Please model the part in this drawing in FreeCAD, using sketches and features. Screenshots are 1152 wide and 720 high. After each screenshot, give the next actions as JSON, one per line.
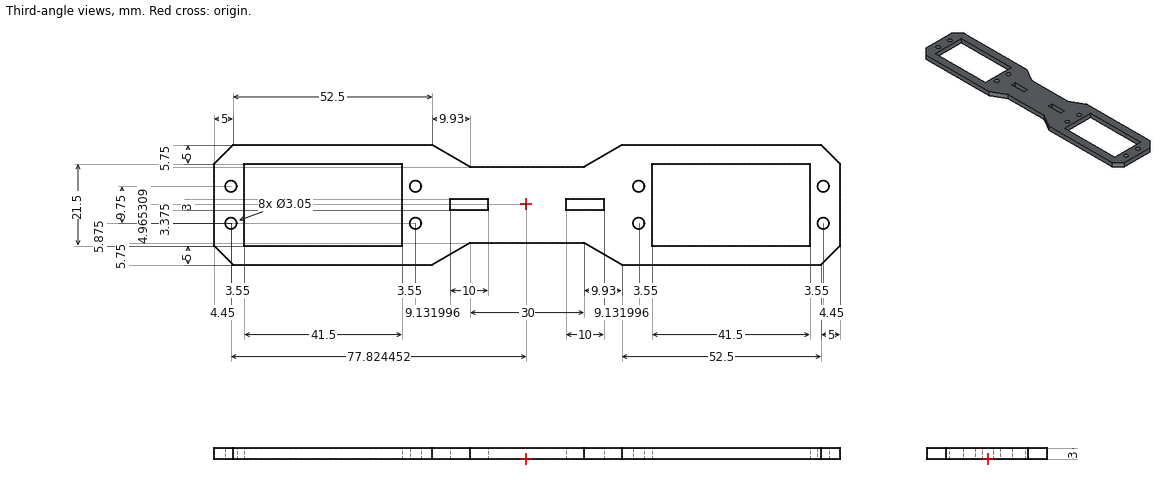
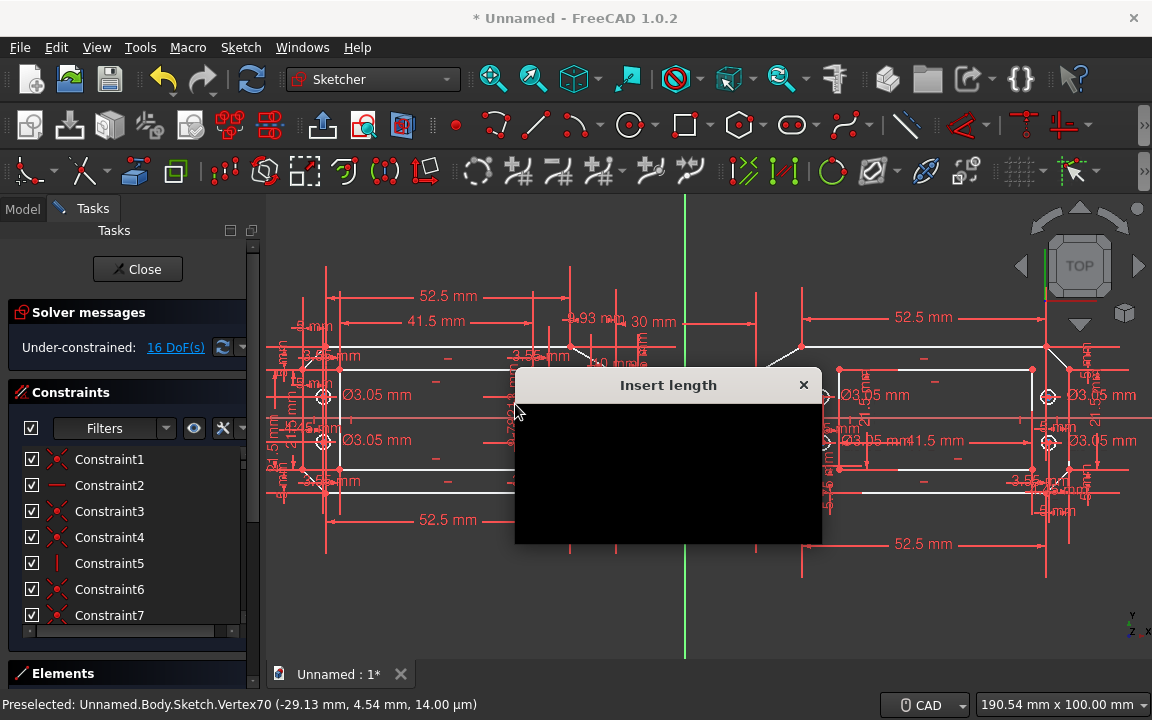
{"action": "type", "text": "9.75"}
{"action": "key", "text": "Return"}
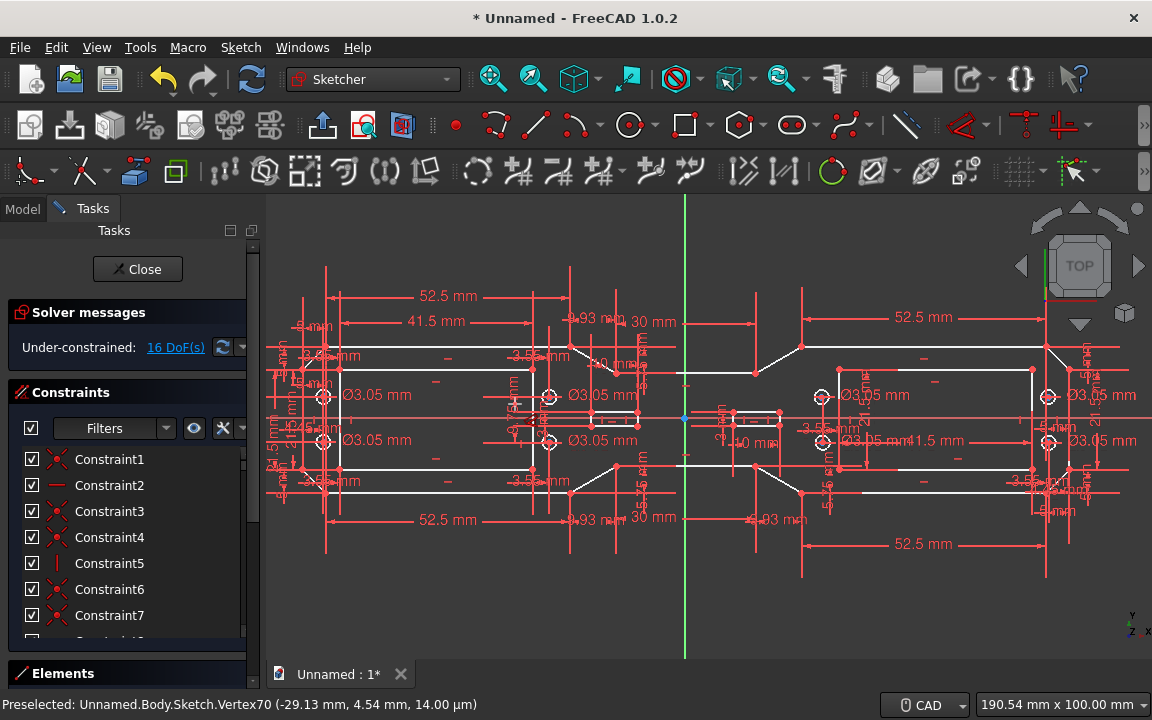
{"action": "scroll", "coordinate": [839, 370], "scroll_direction": "up", "scroll_amount": 5}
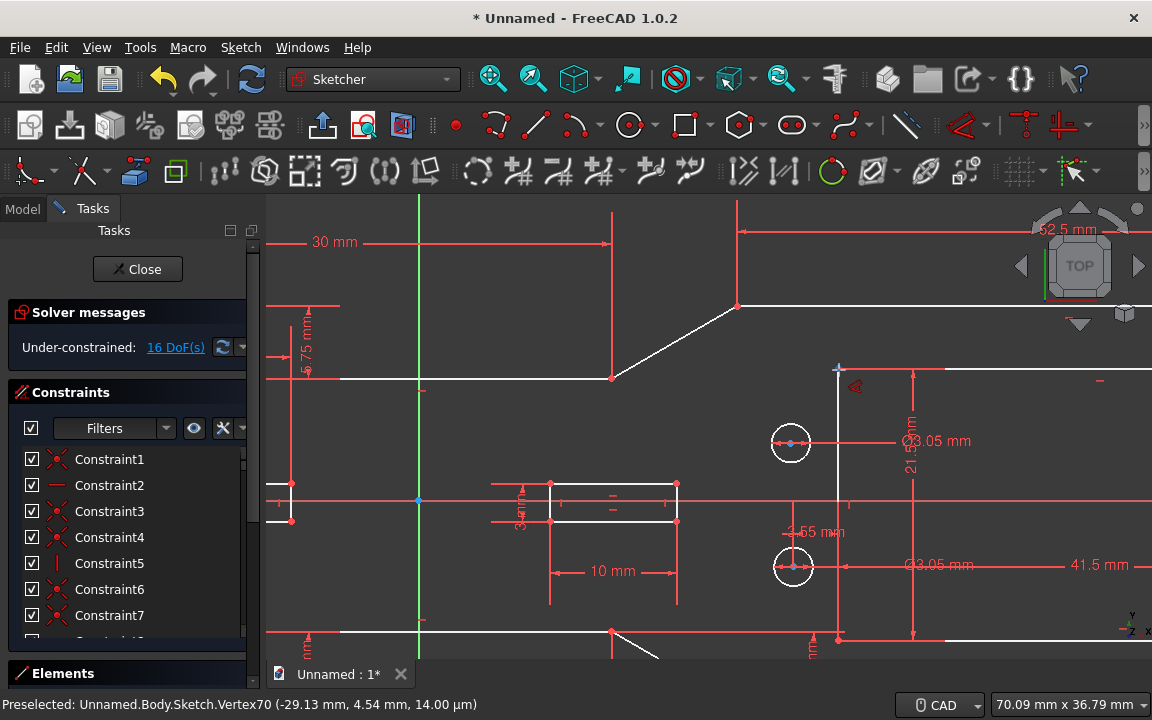
{"action": "left_click", "coordinate": [838, 369]}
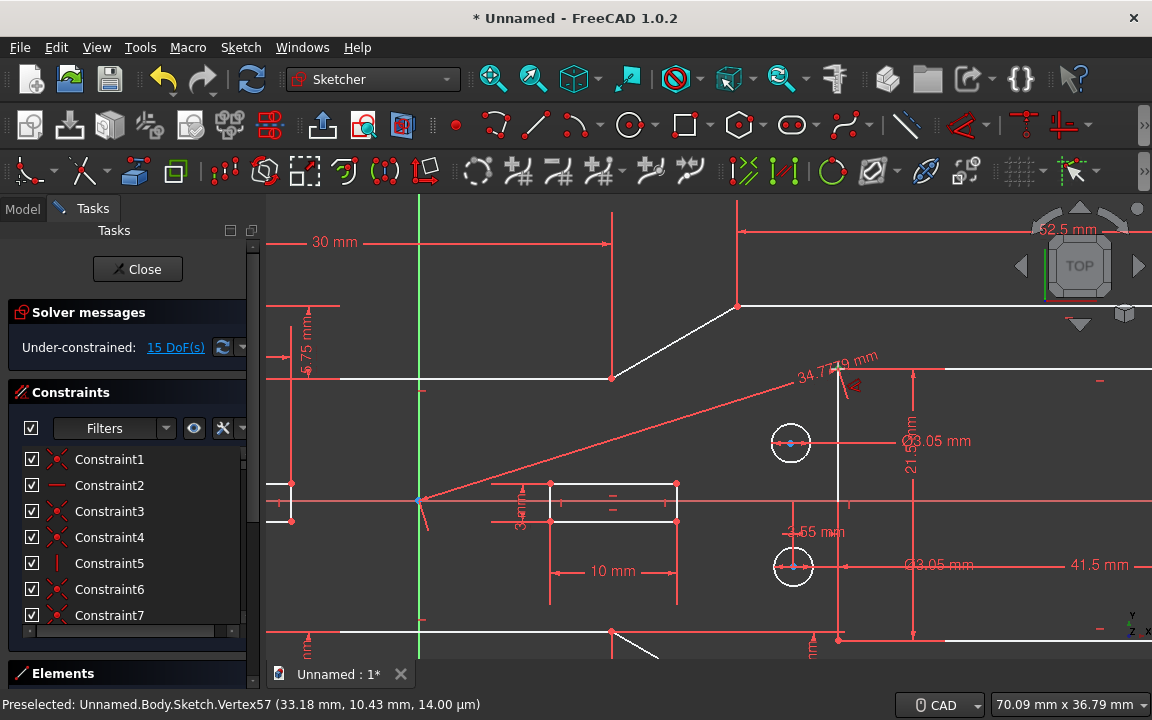
{"action": "left_click", "coordinate": [791, 443]}
{"action": "left_click", "coordinate": [815, 335]}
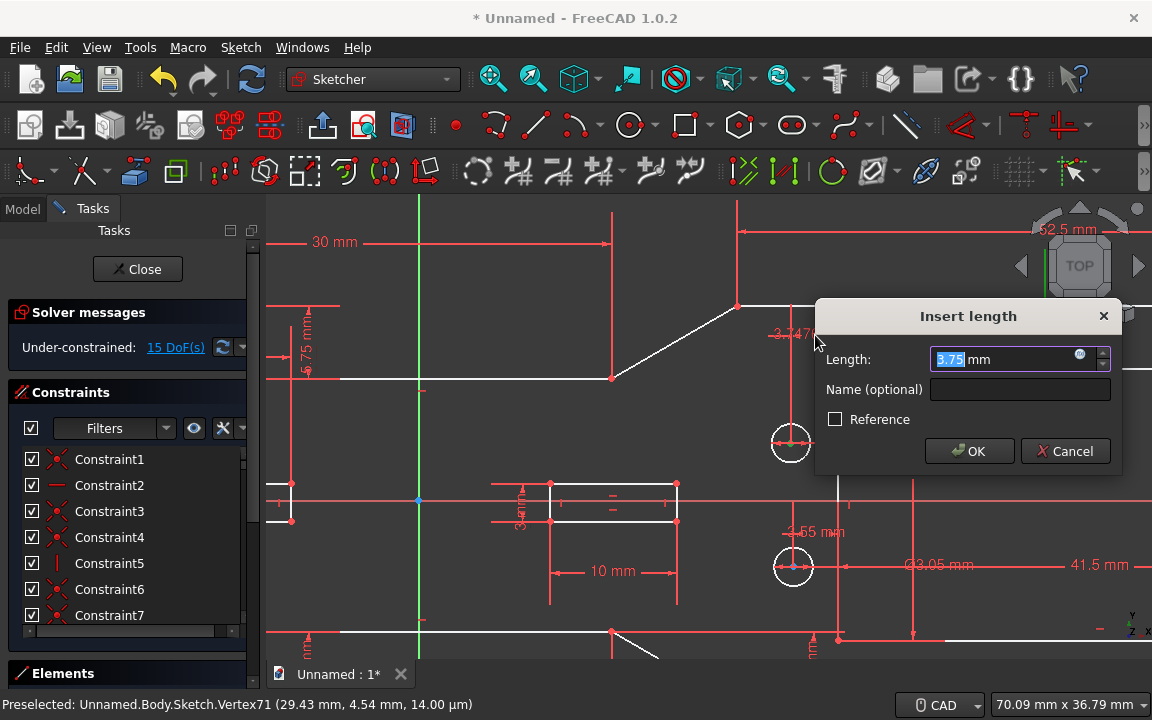
{"action": "type", "text": "3.55"}
{"action": "key", "text": "Return"}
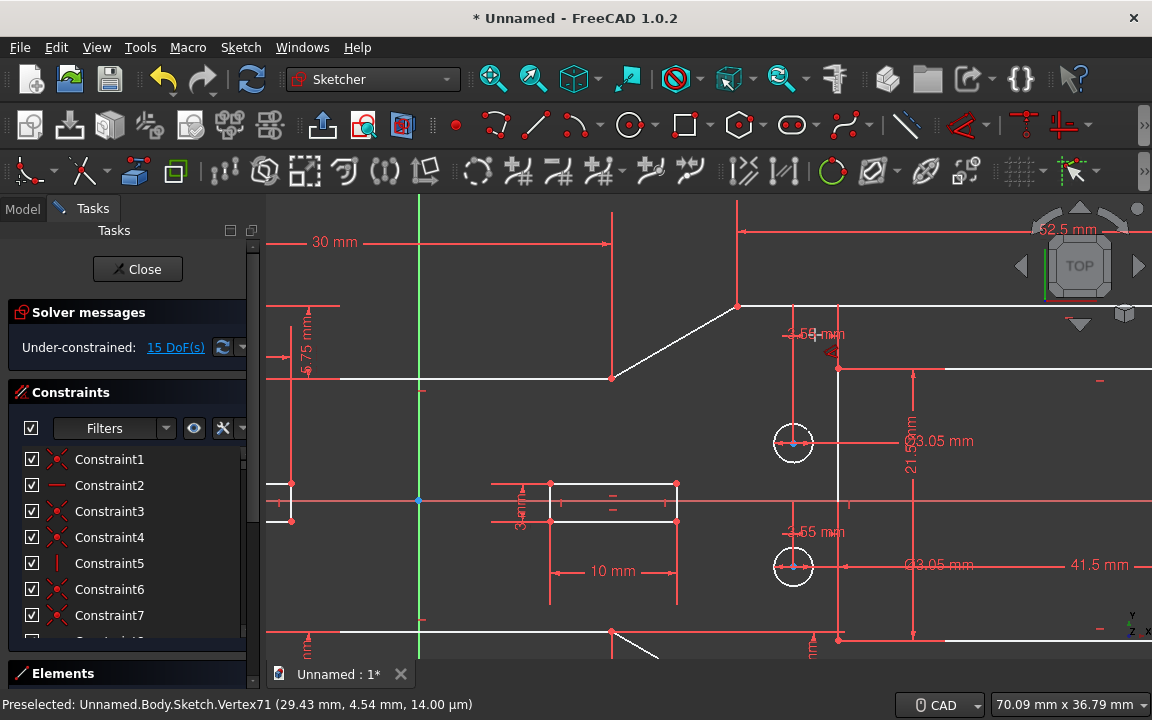
{"action": "scroll", "coordinate": [712, 402], "scroll_direction": "down", "scroll_amount": 7}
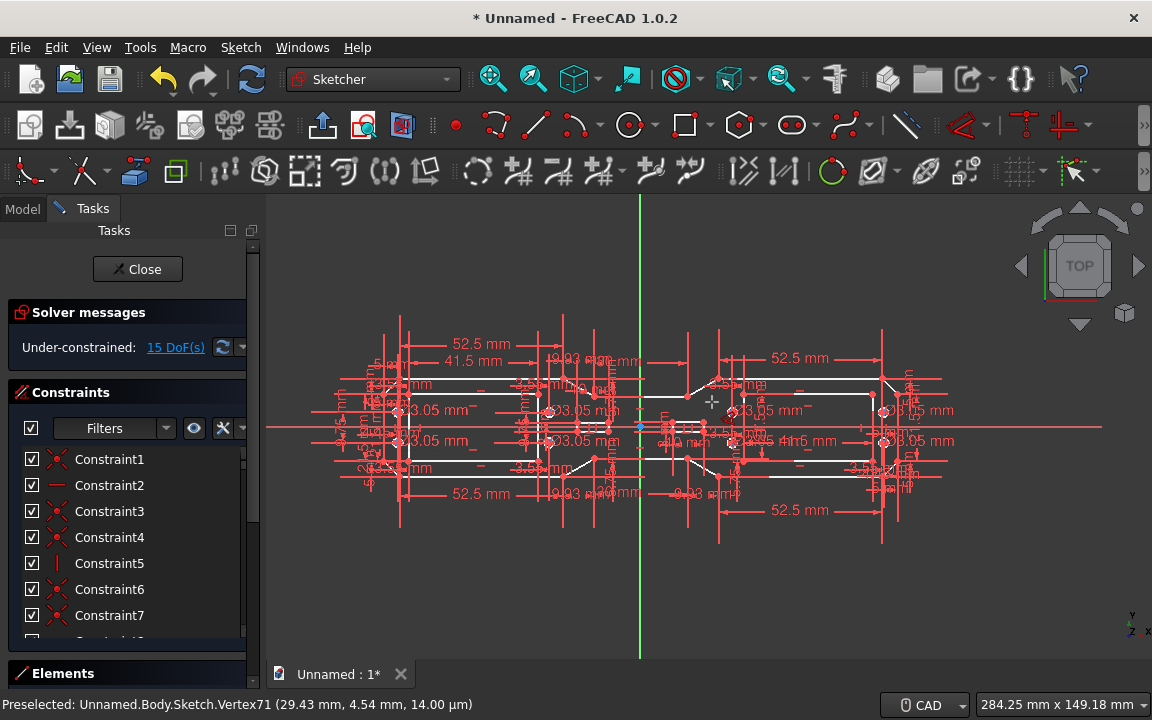
{"action": "scroll", "coordinate": [732, 443], "scroll_direction": "up", "scroll_amount": 2}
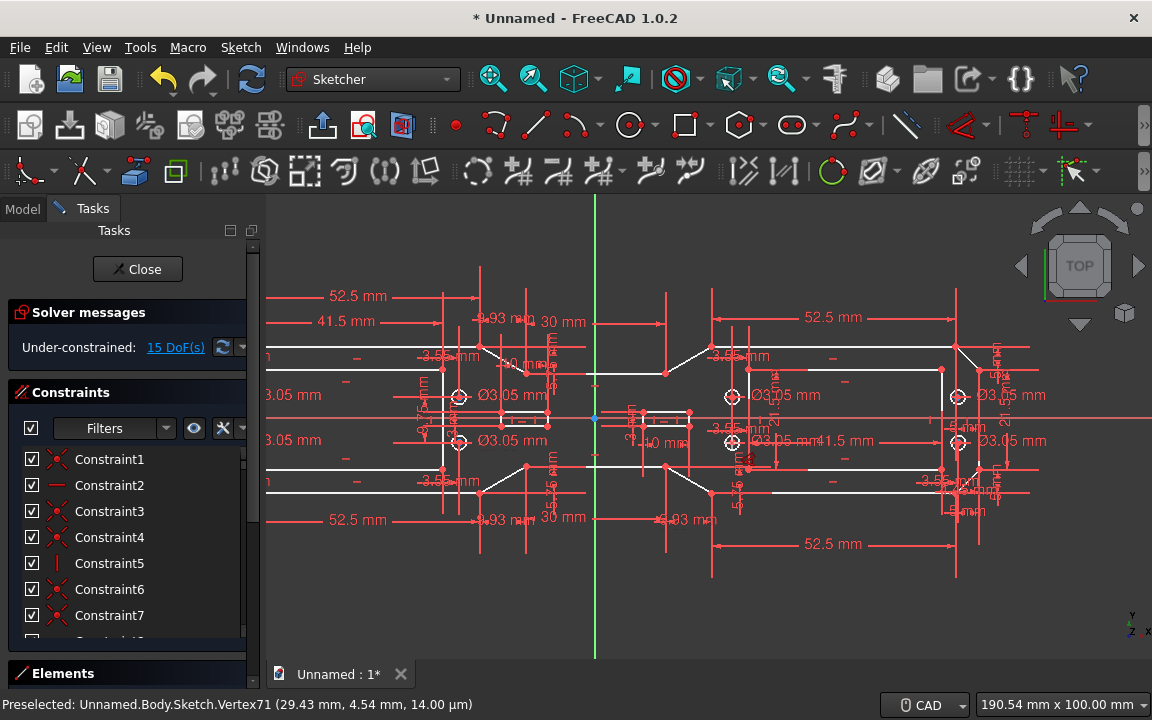
{"action": "left_click", "coordinate": [732, 443]}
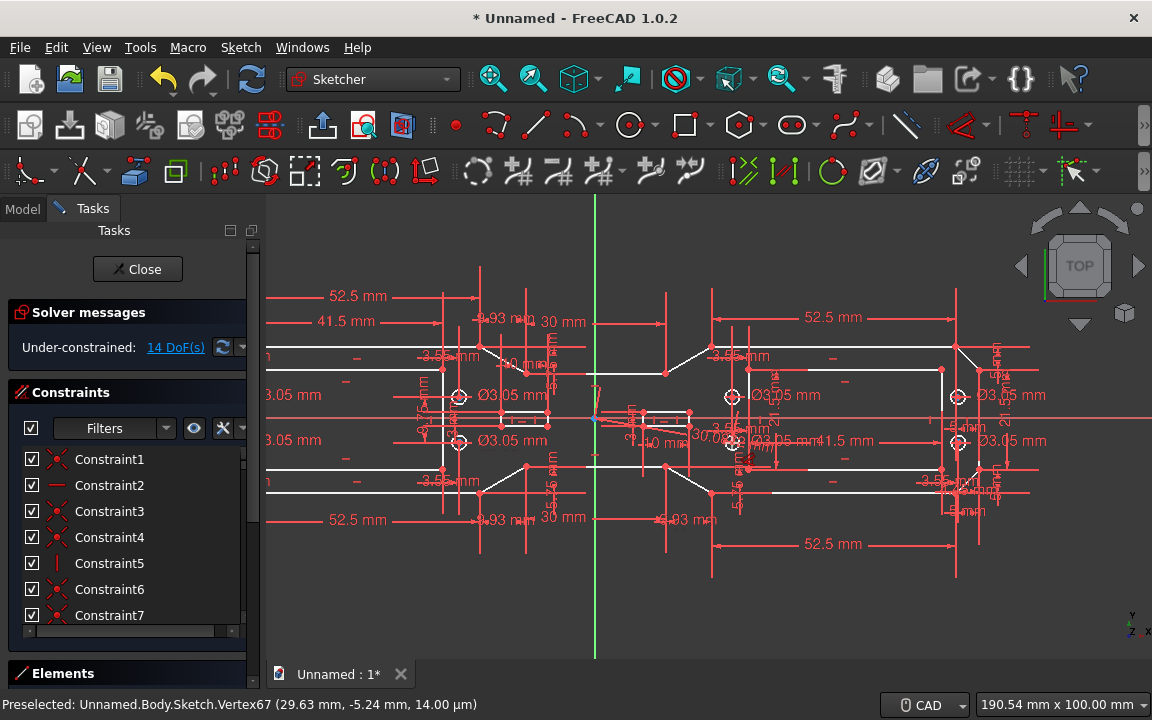
{"action": "left_click", "coordinate": [732, 397]}
{"action": "left_click", "coordinate": [862, 404]}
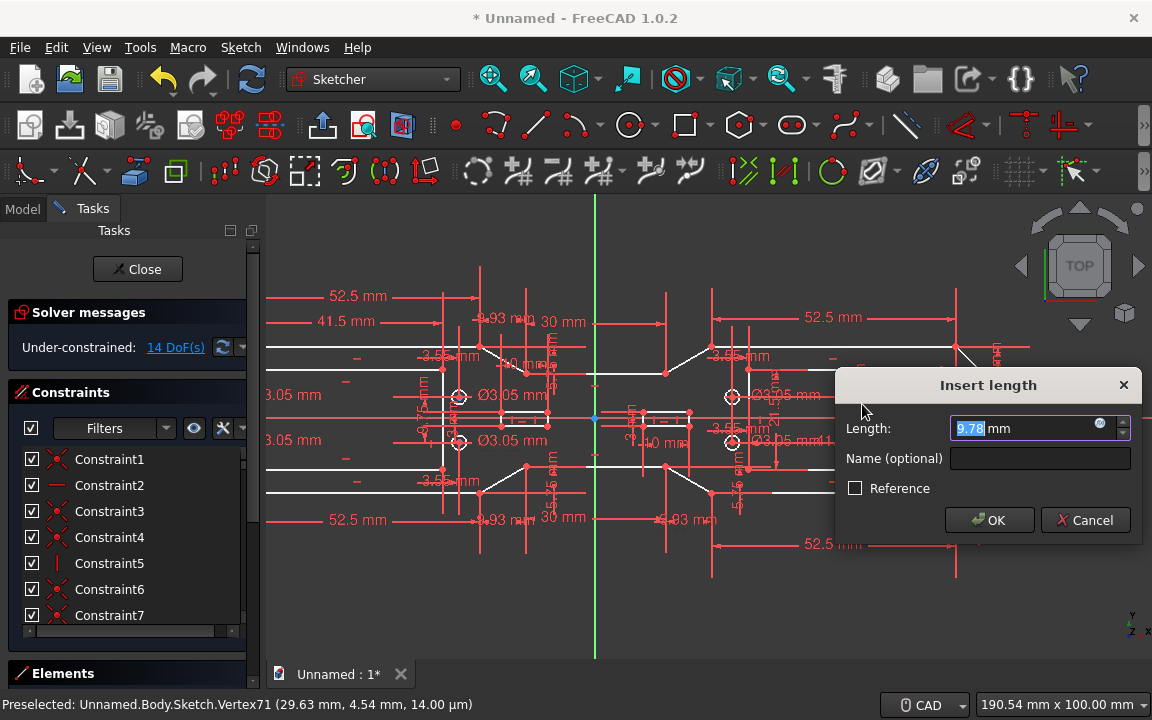
{"action": "type", "text": "9.75"}
{"action": "key", "text": "Return"}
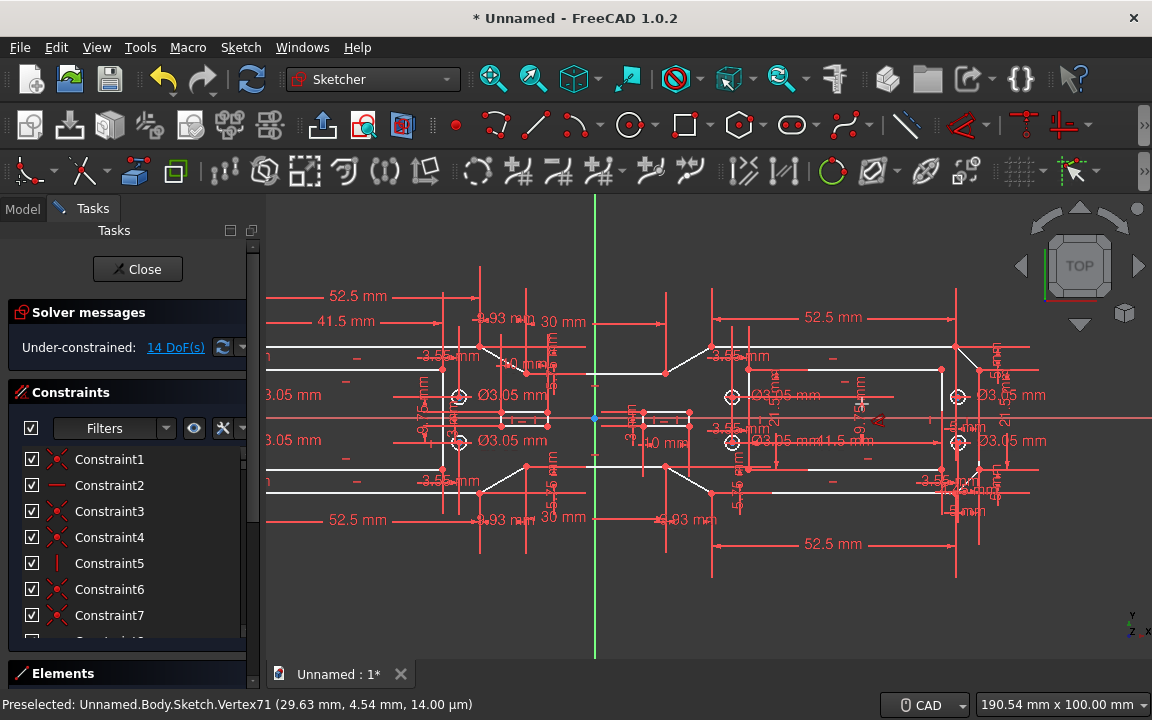
{"action": "scroll", "coordinate": [942, 370], "scroll_direction": "up", "scroll_amount": 5}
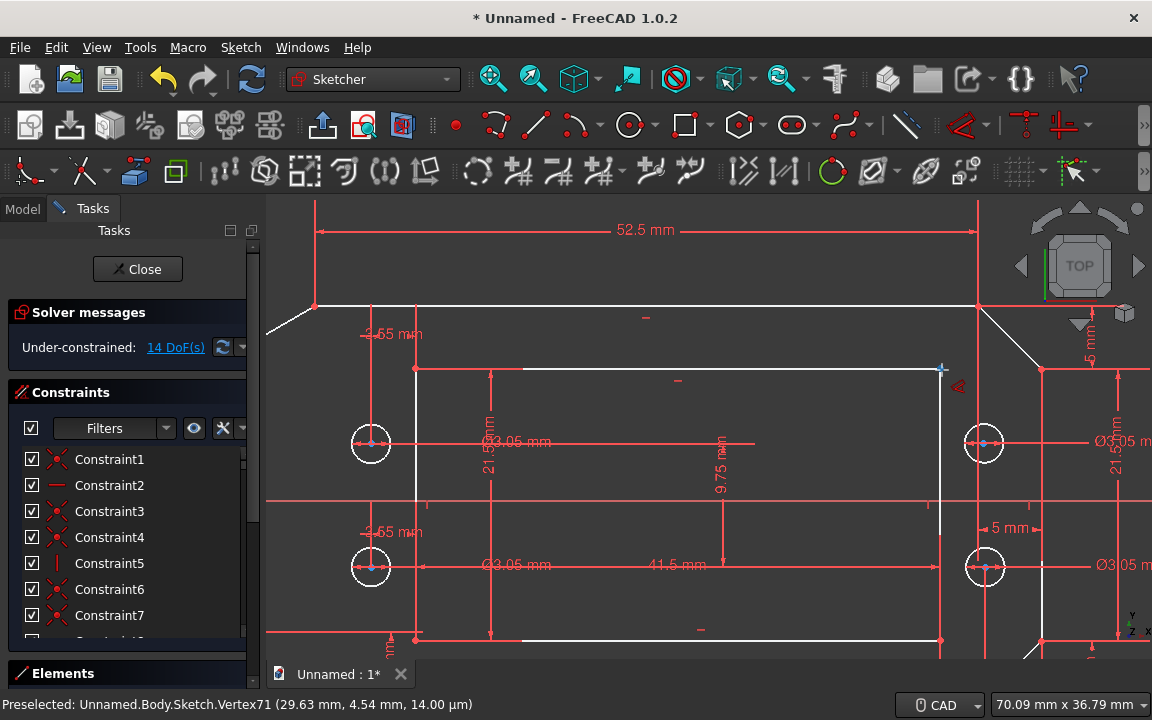
{"action": "left_click", "coordinate": [940, 369]}